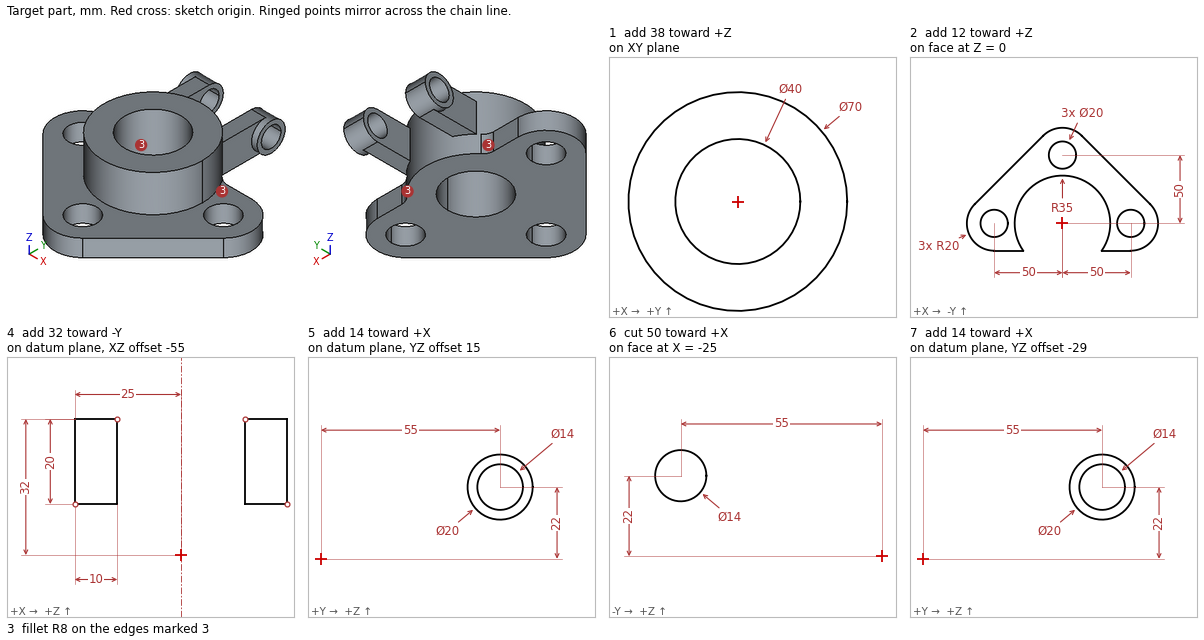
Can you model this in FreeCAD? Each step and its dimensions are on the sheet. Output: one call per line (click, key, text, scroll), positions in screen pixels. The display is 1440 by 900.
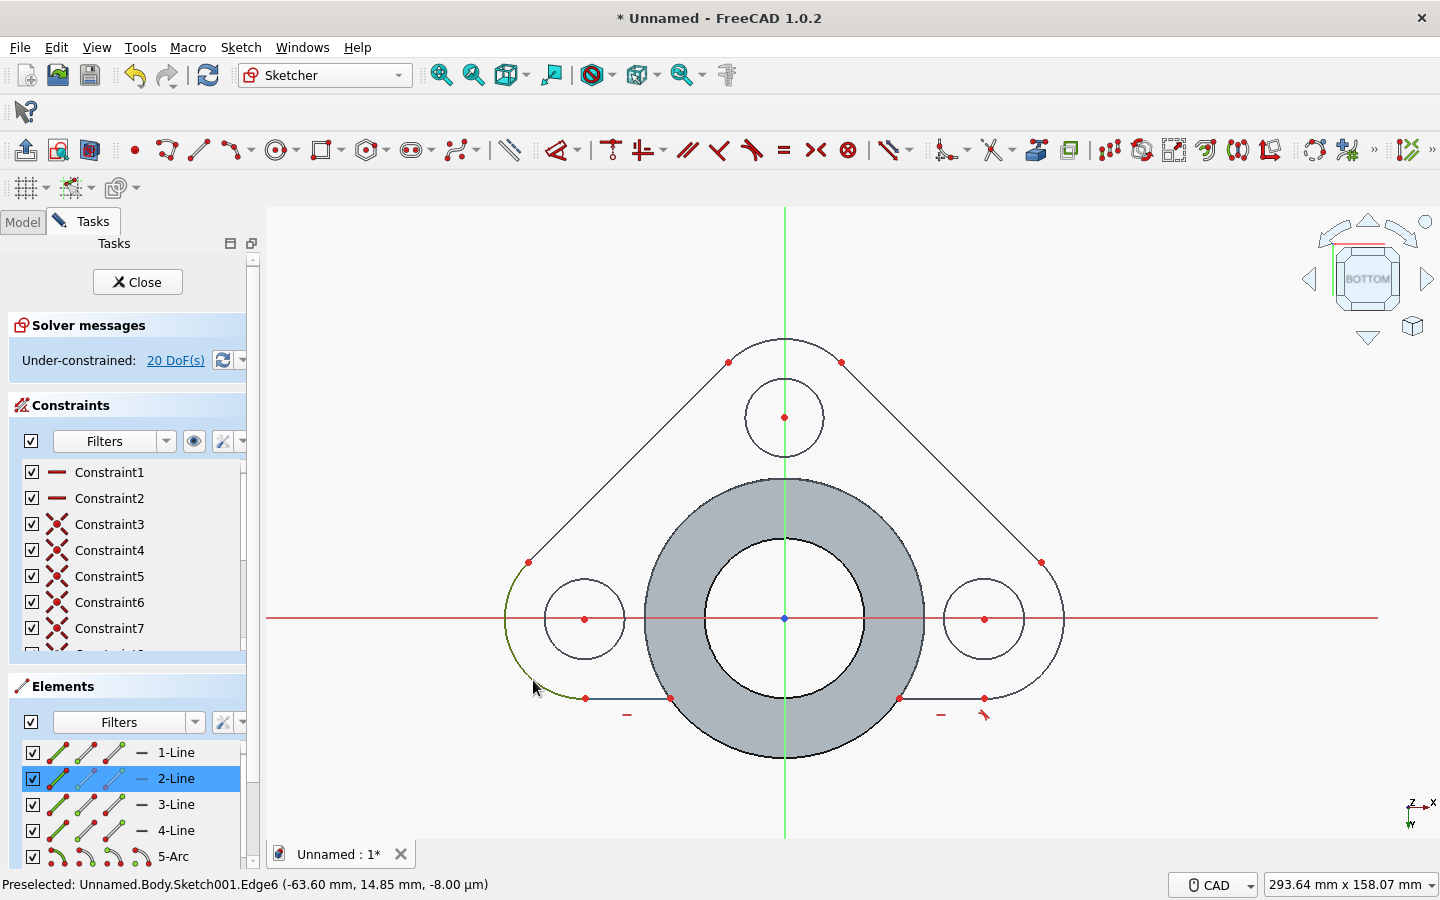
key(t)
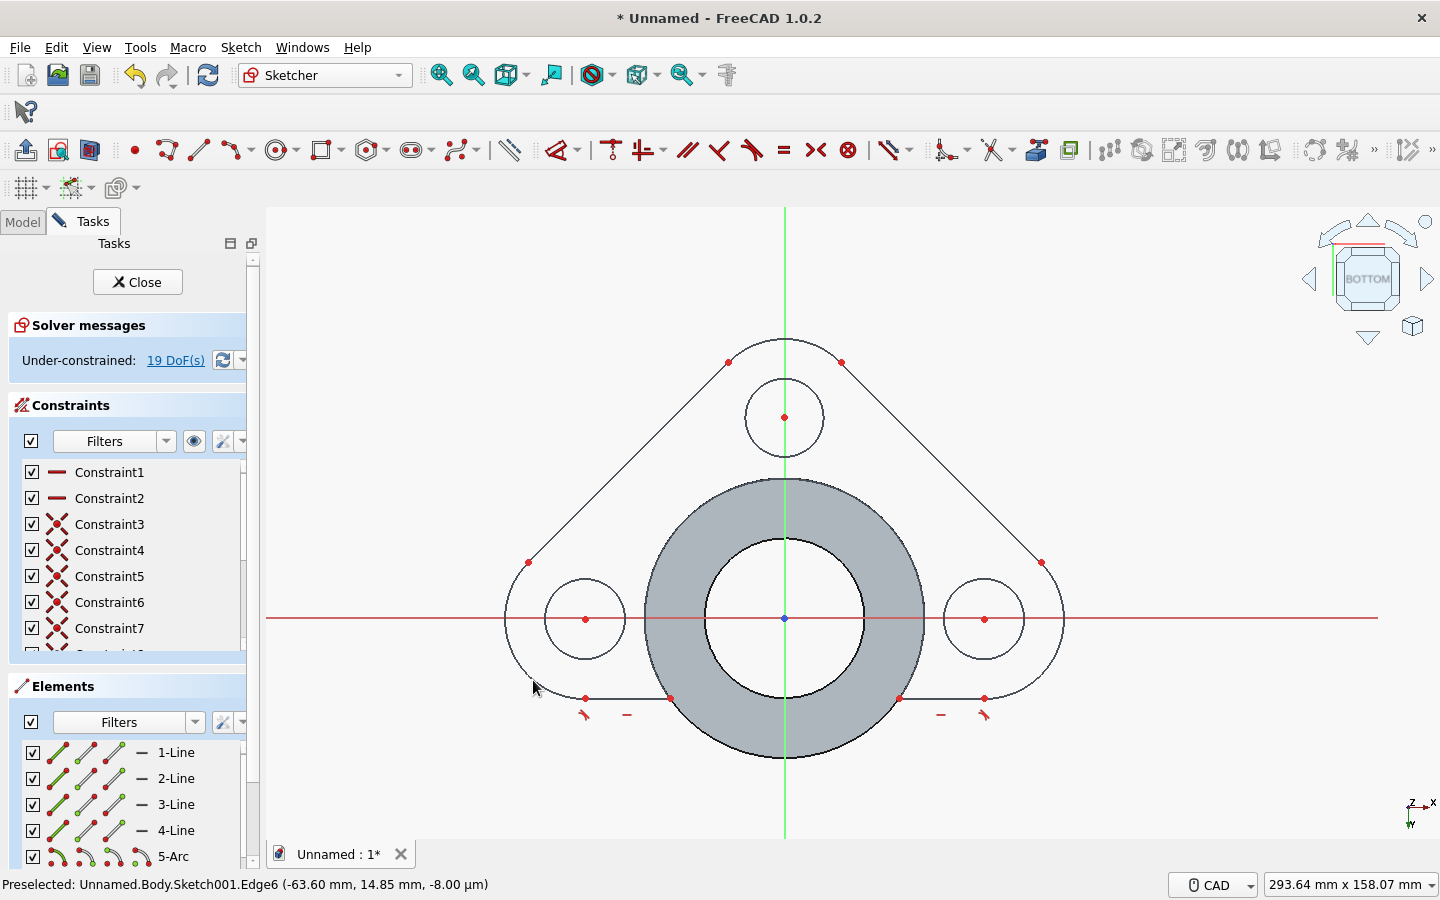
click(588, 503)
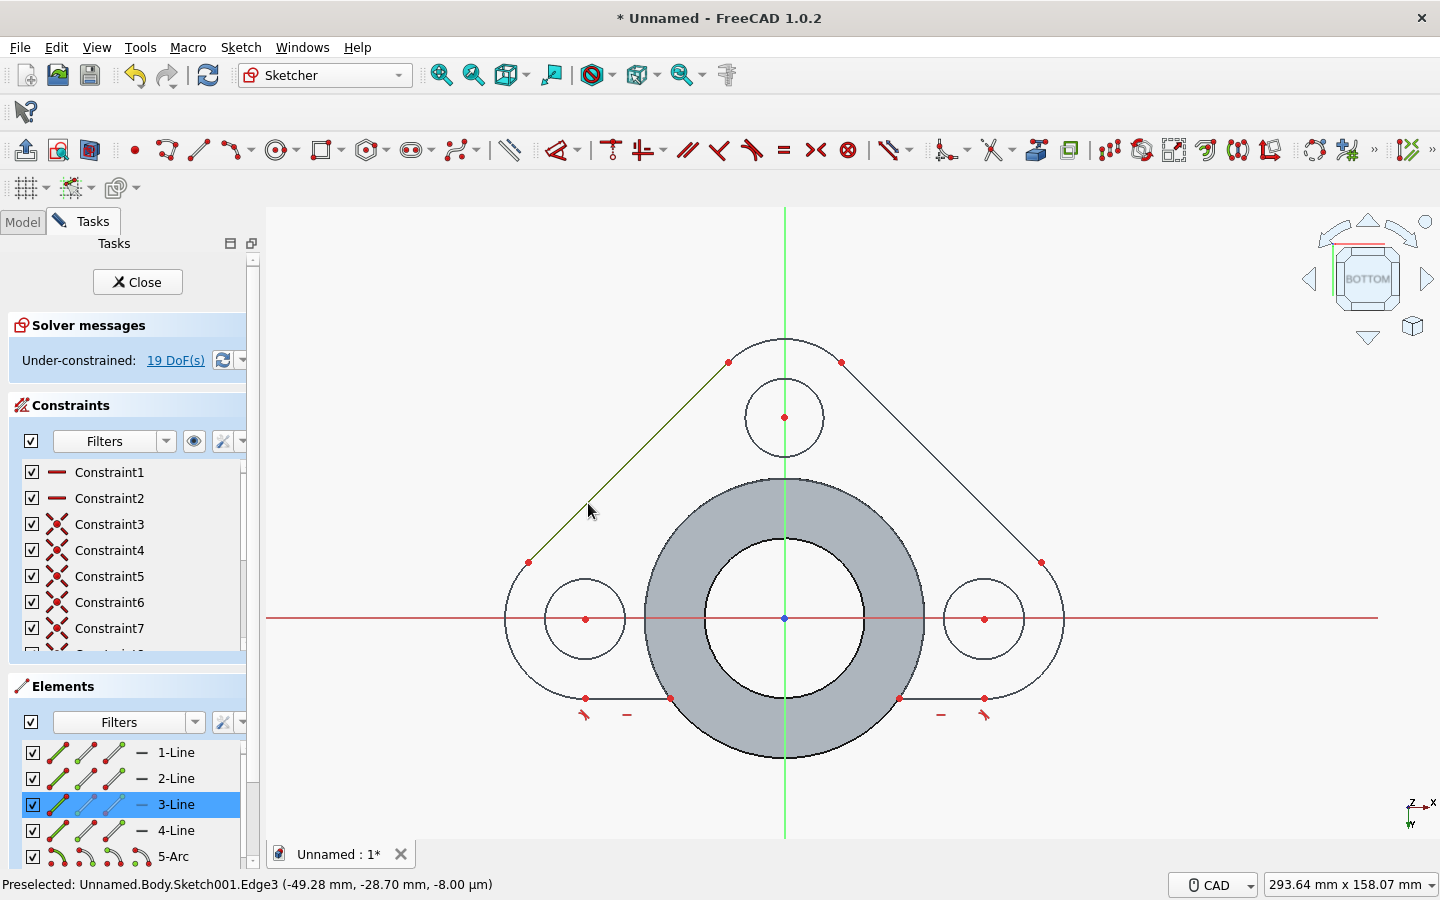
click(533, 680)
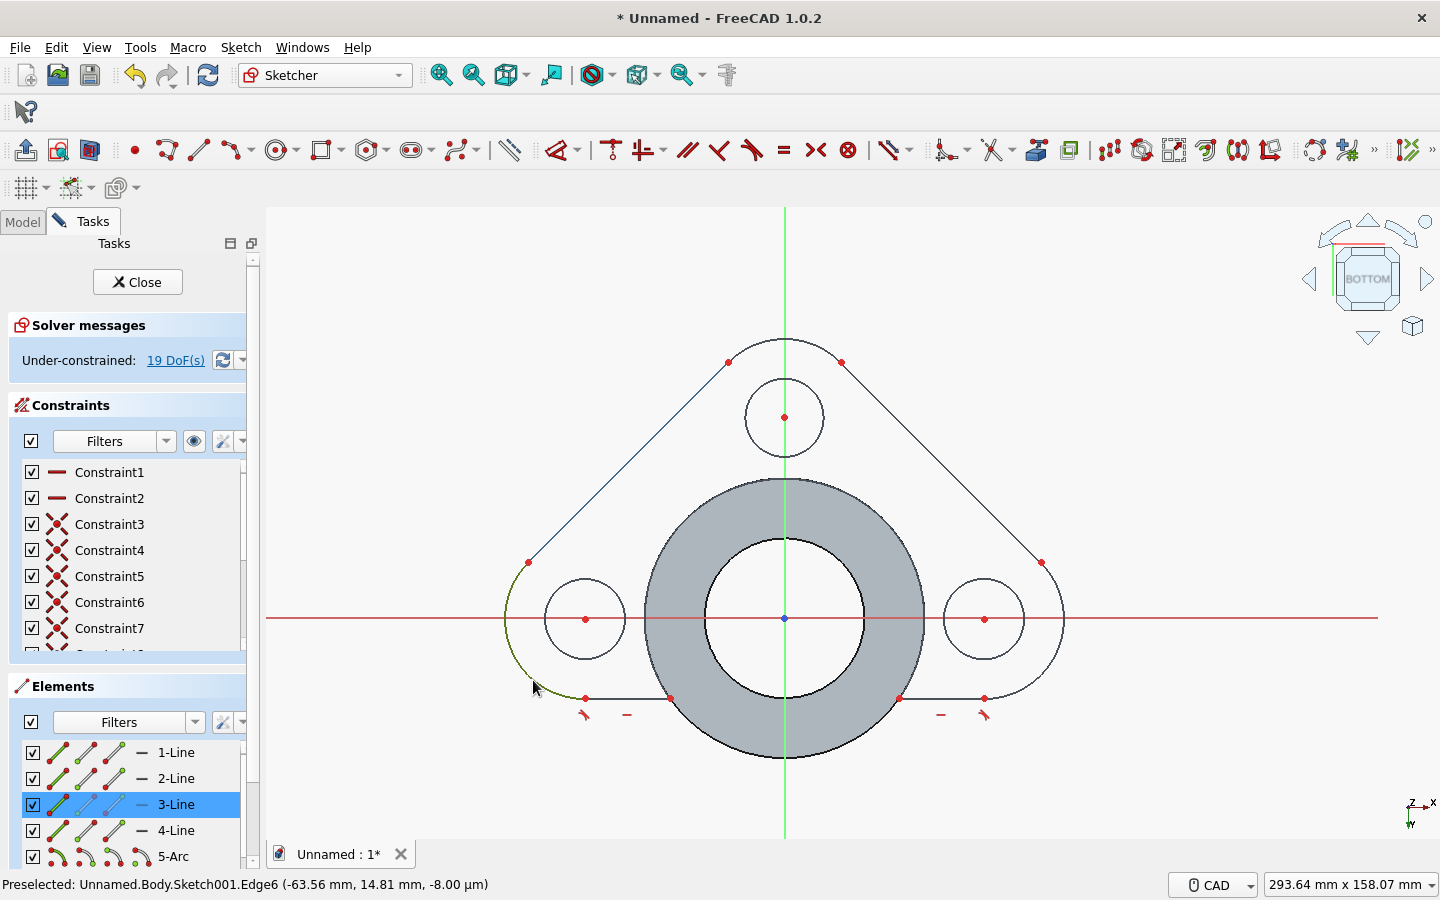
click(752, 150)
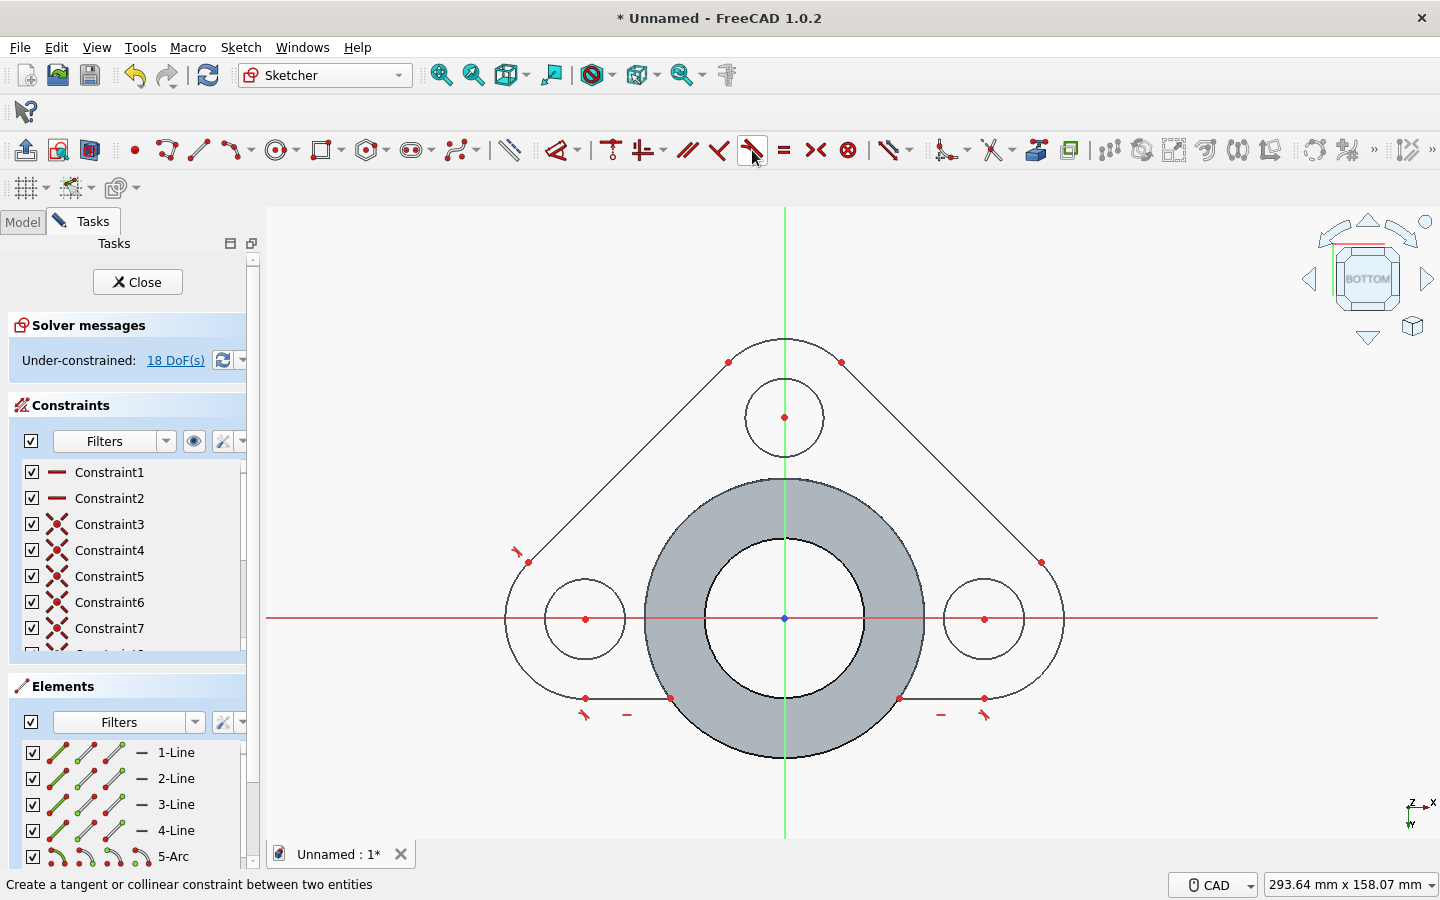
click(588, 503)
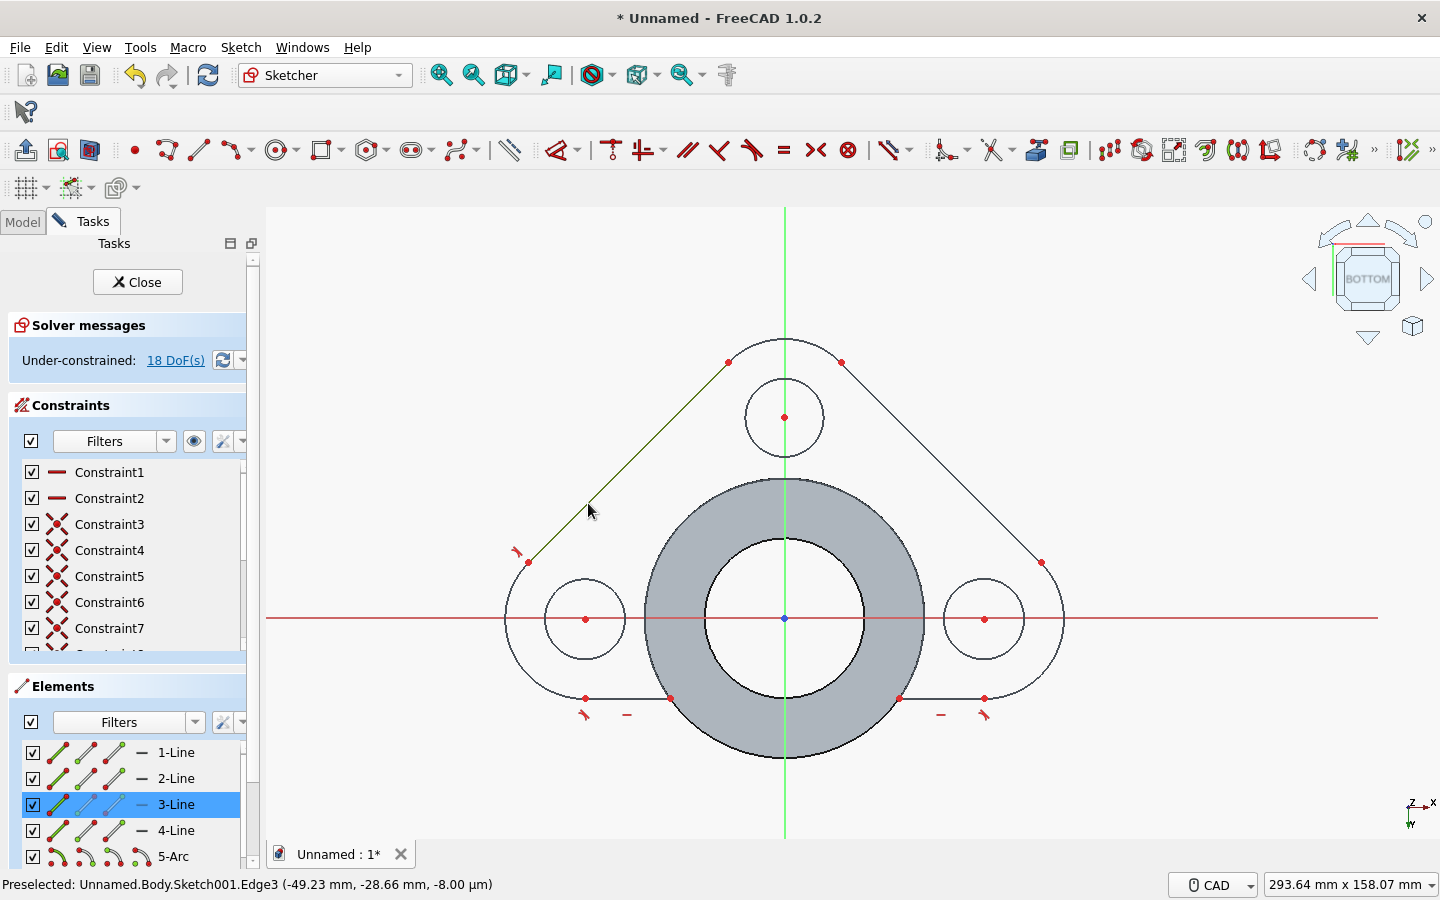
click(809, 343)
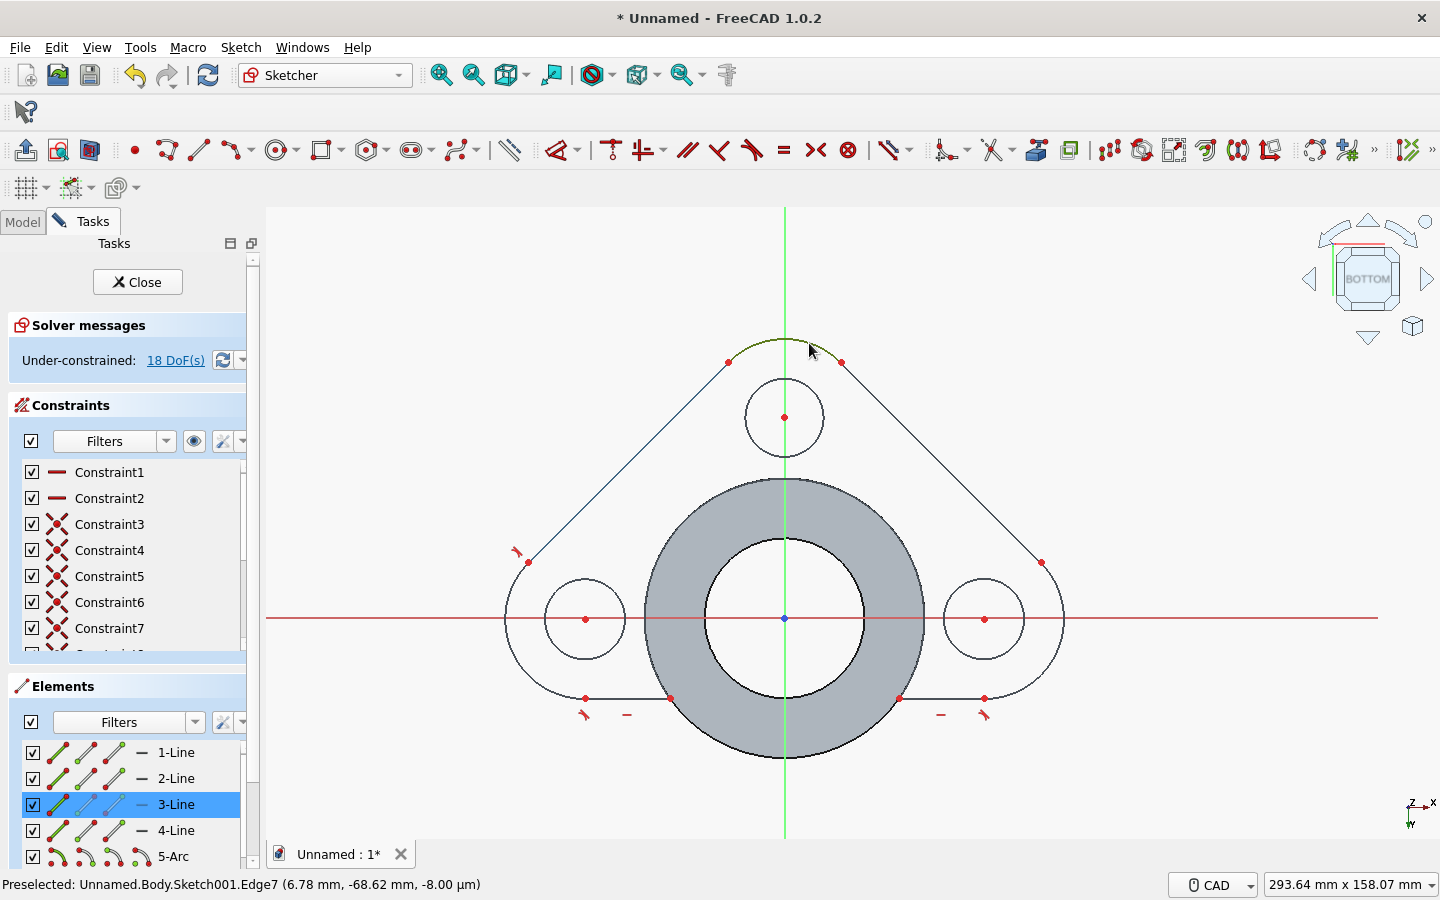
click(752, 150)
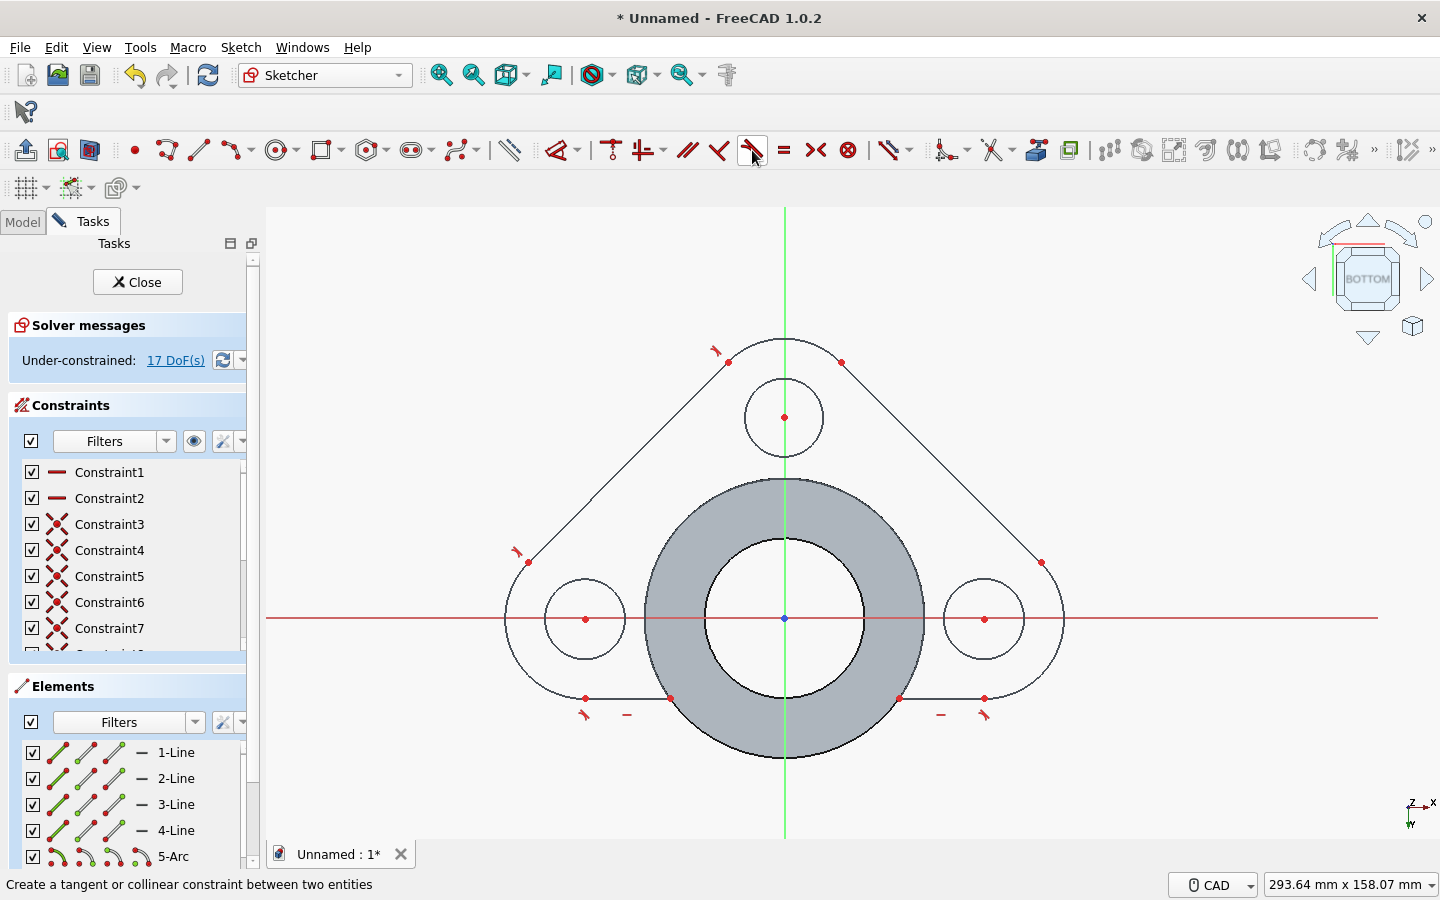
click(901, 423)